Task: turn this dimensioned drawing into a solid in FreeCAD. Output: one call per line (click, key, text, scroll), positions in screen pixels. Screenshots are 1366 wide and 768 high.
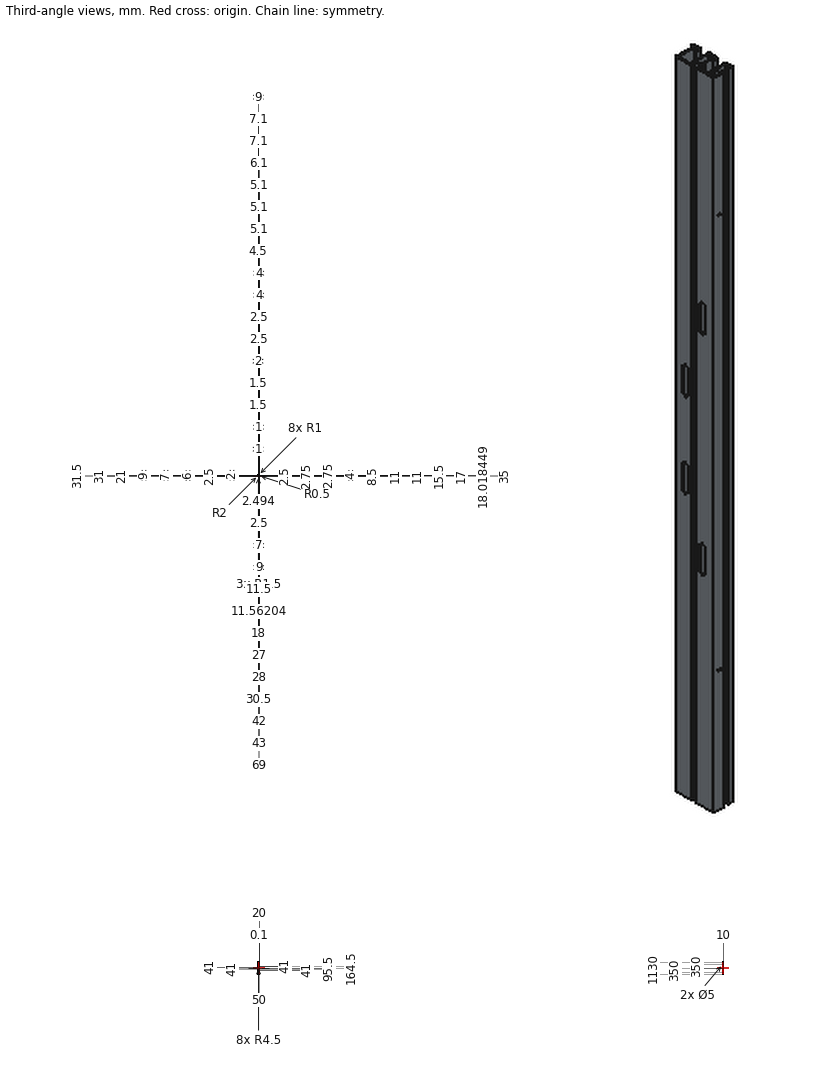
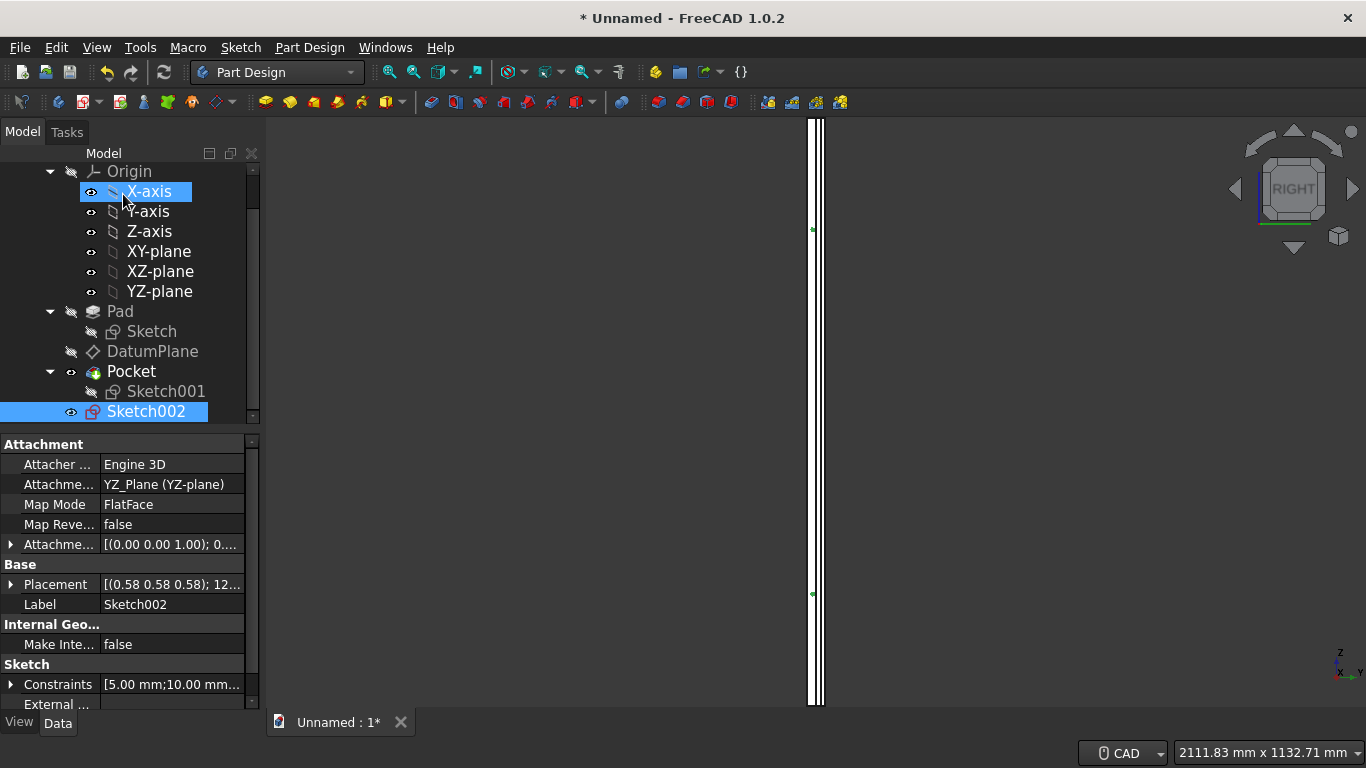
click(432, 102)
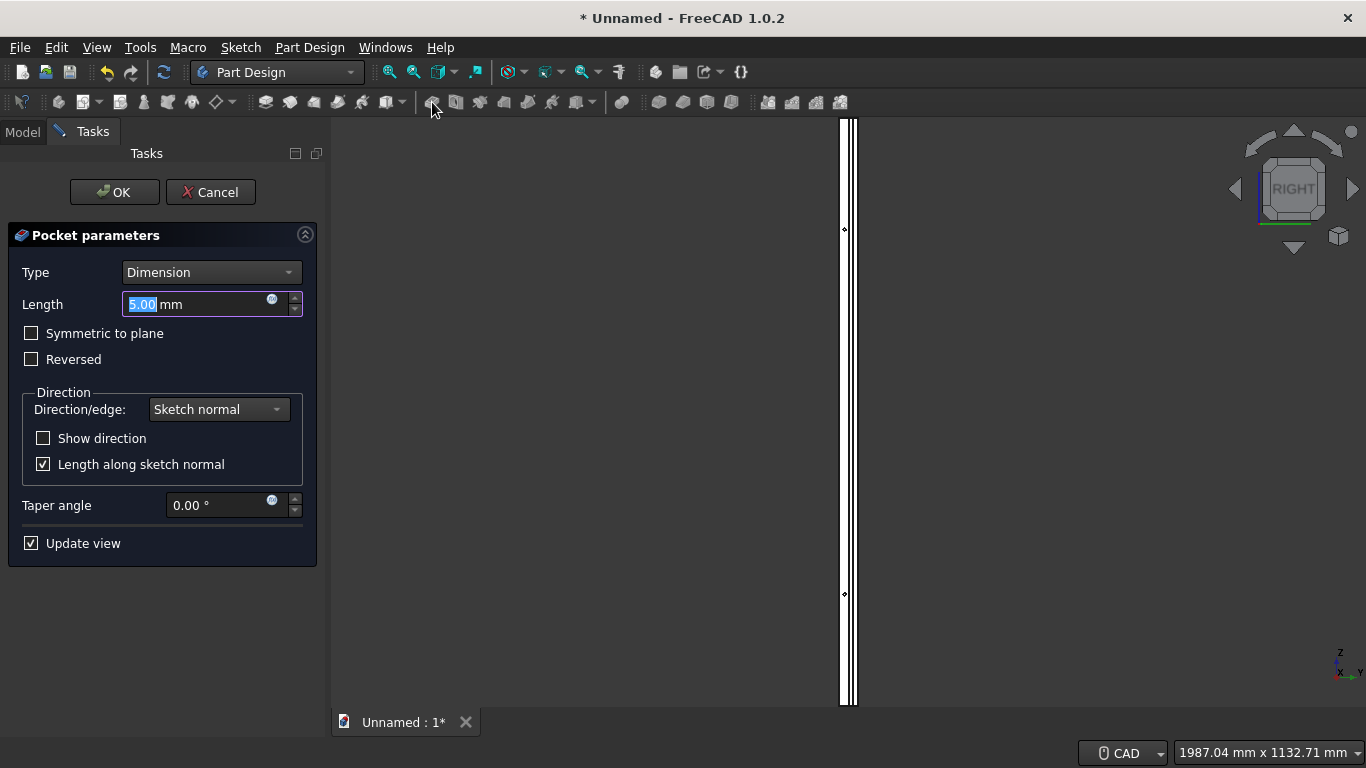
text(0.1)
key(Tab)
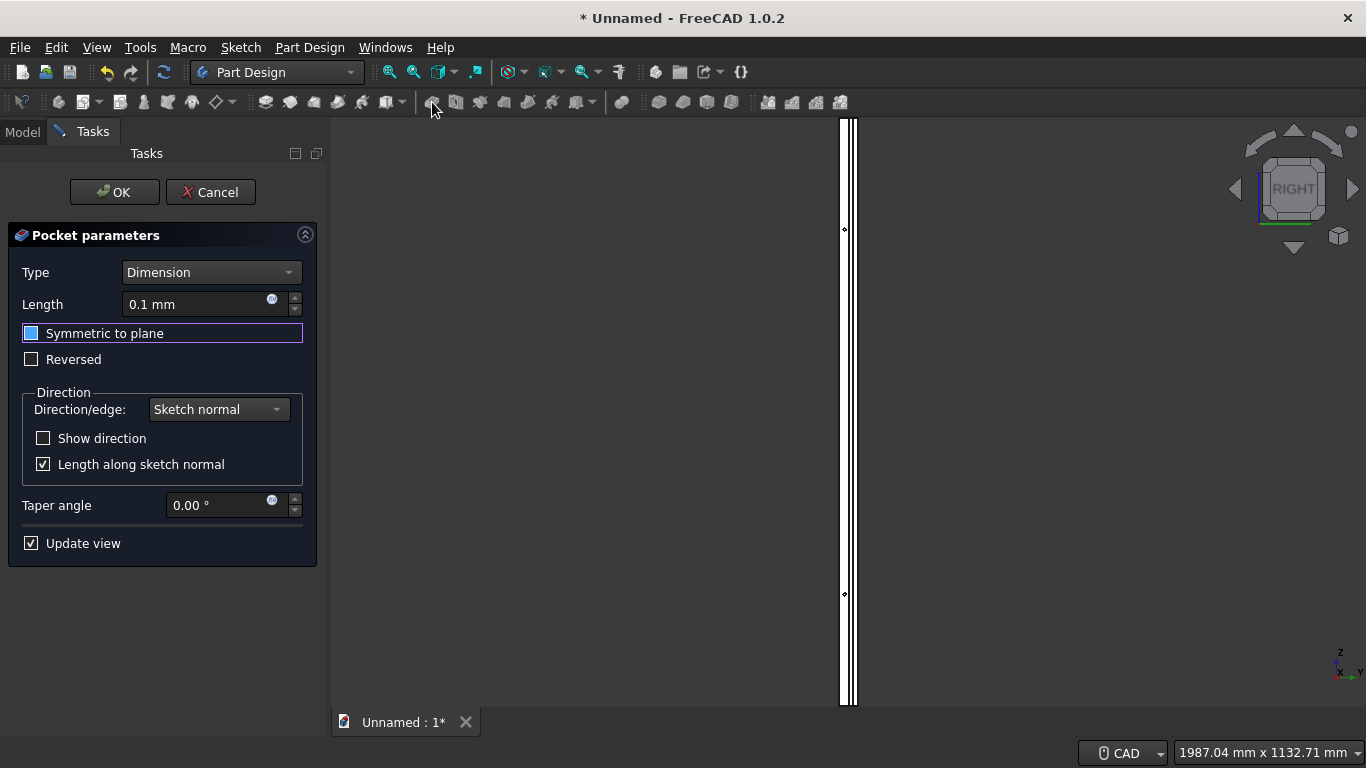
click(115, 192)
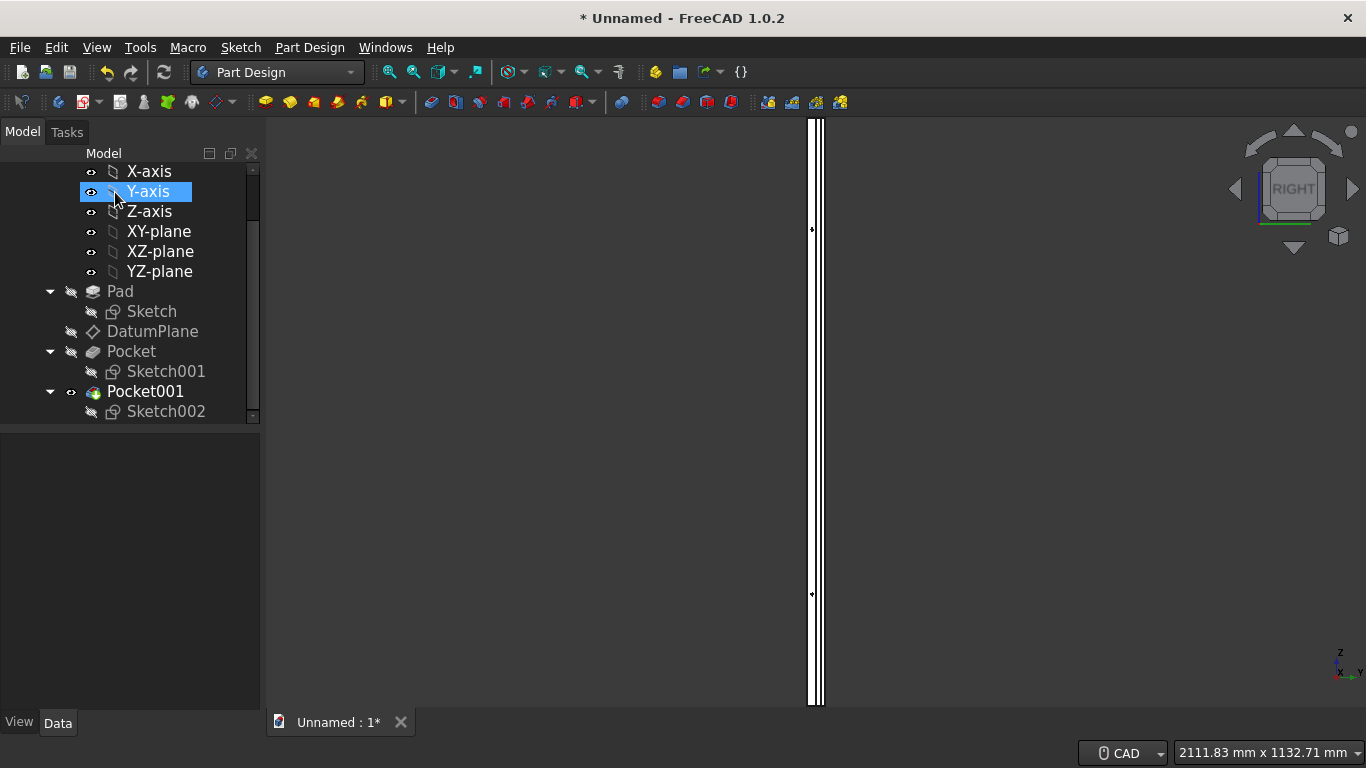
key(0)